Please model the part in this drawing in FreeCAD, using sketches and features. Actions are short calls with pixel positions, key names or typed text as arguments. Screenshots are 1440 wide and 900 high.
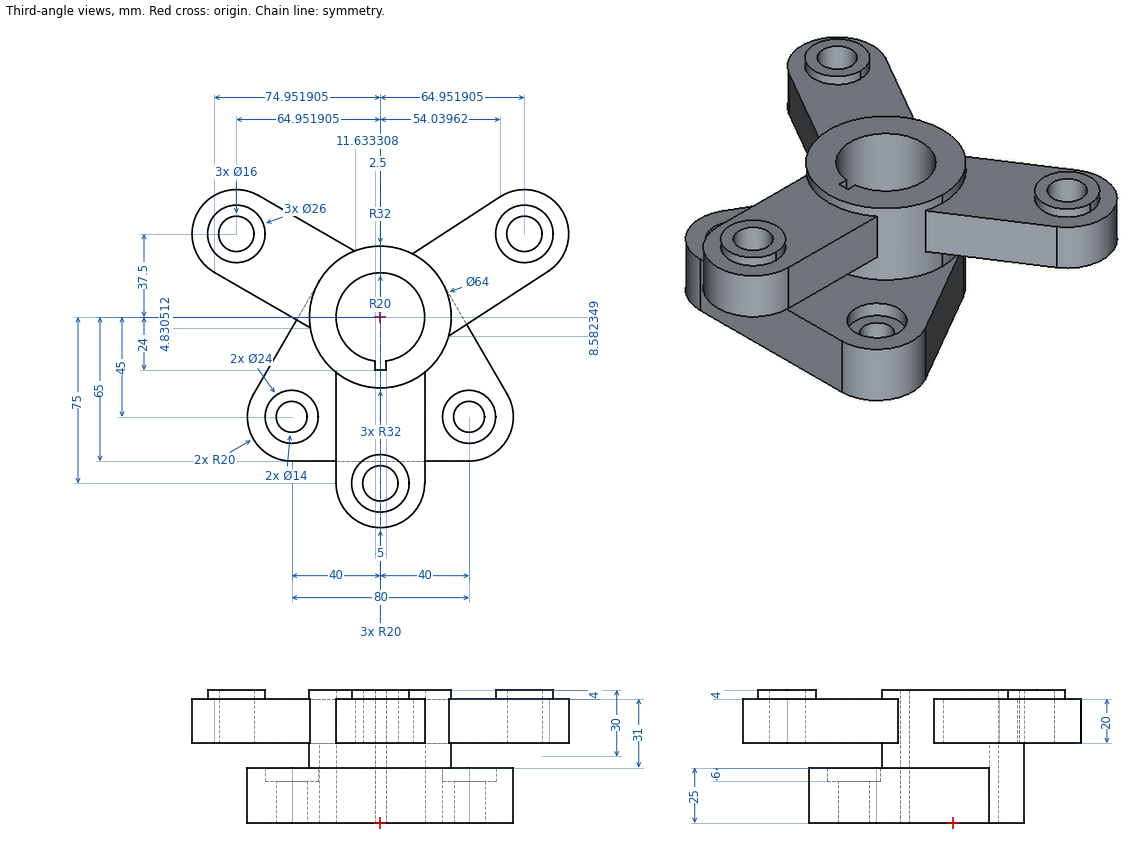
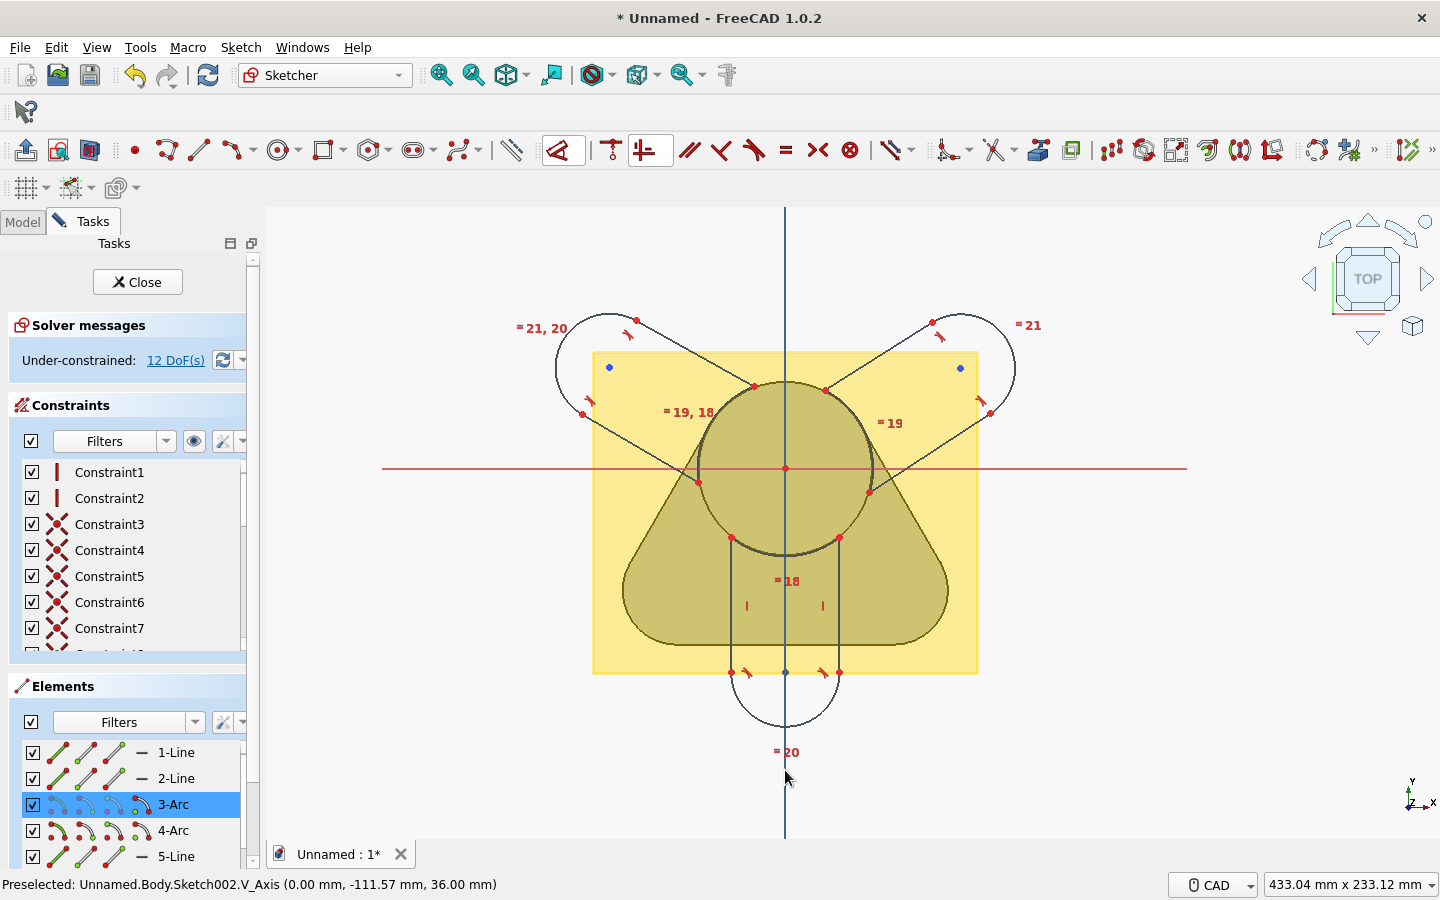
click(612, 150)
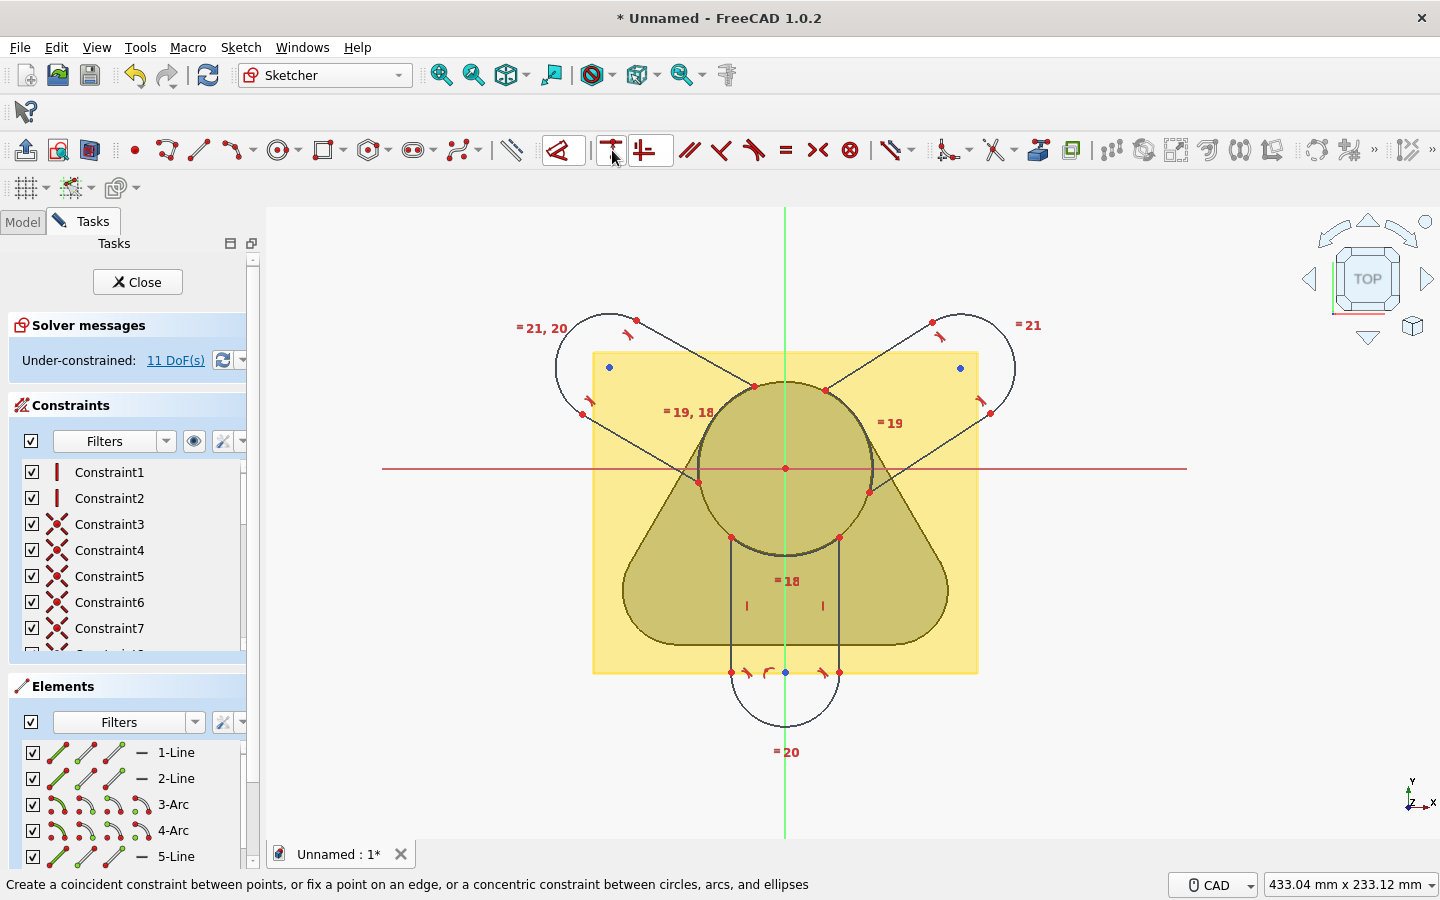
click(610, 368)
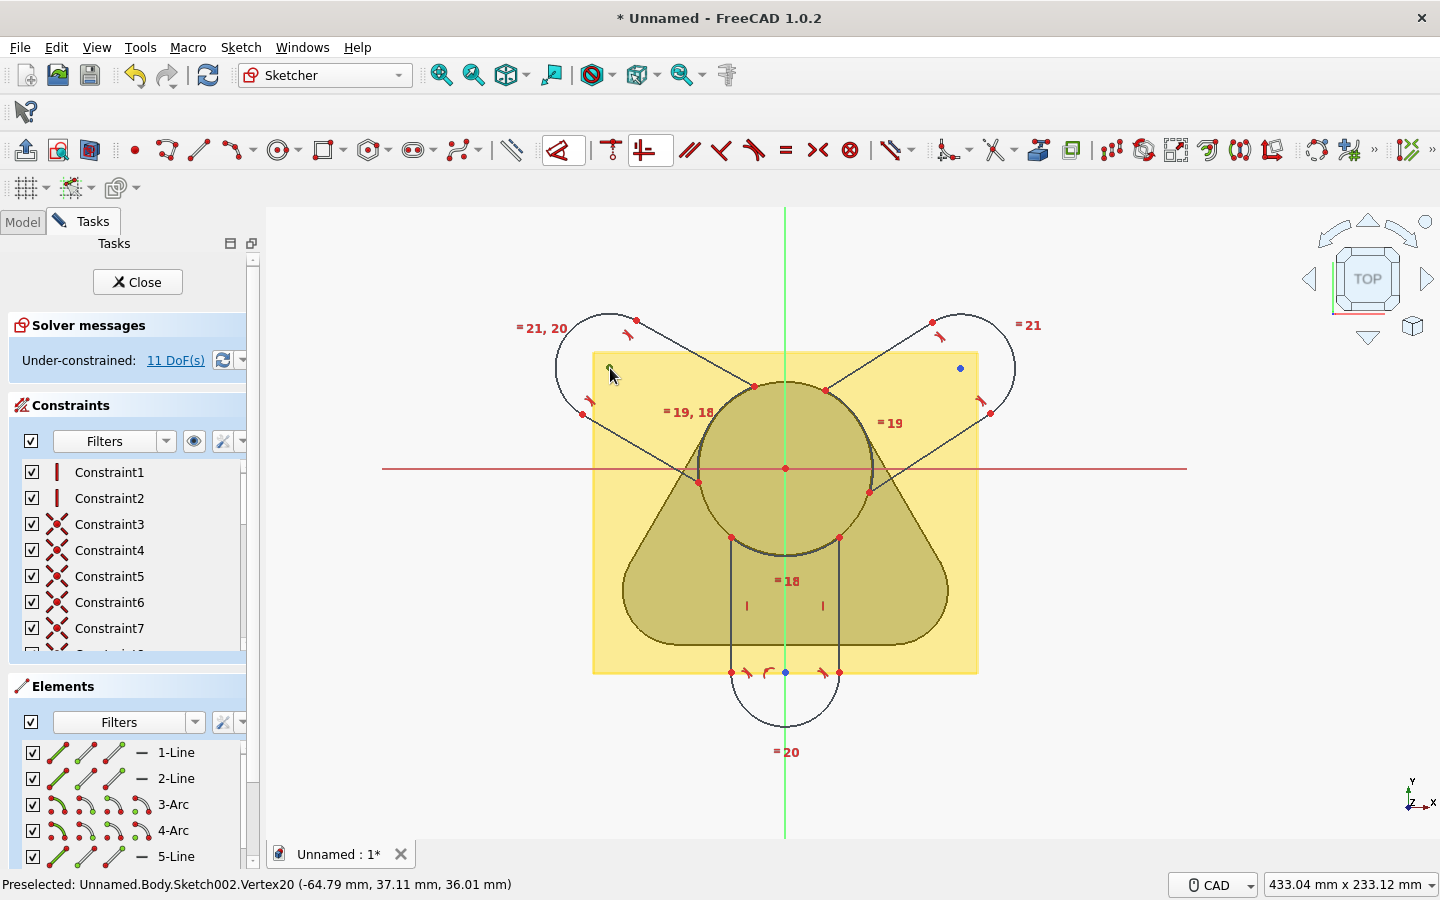
click(961, 368)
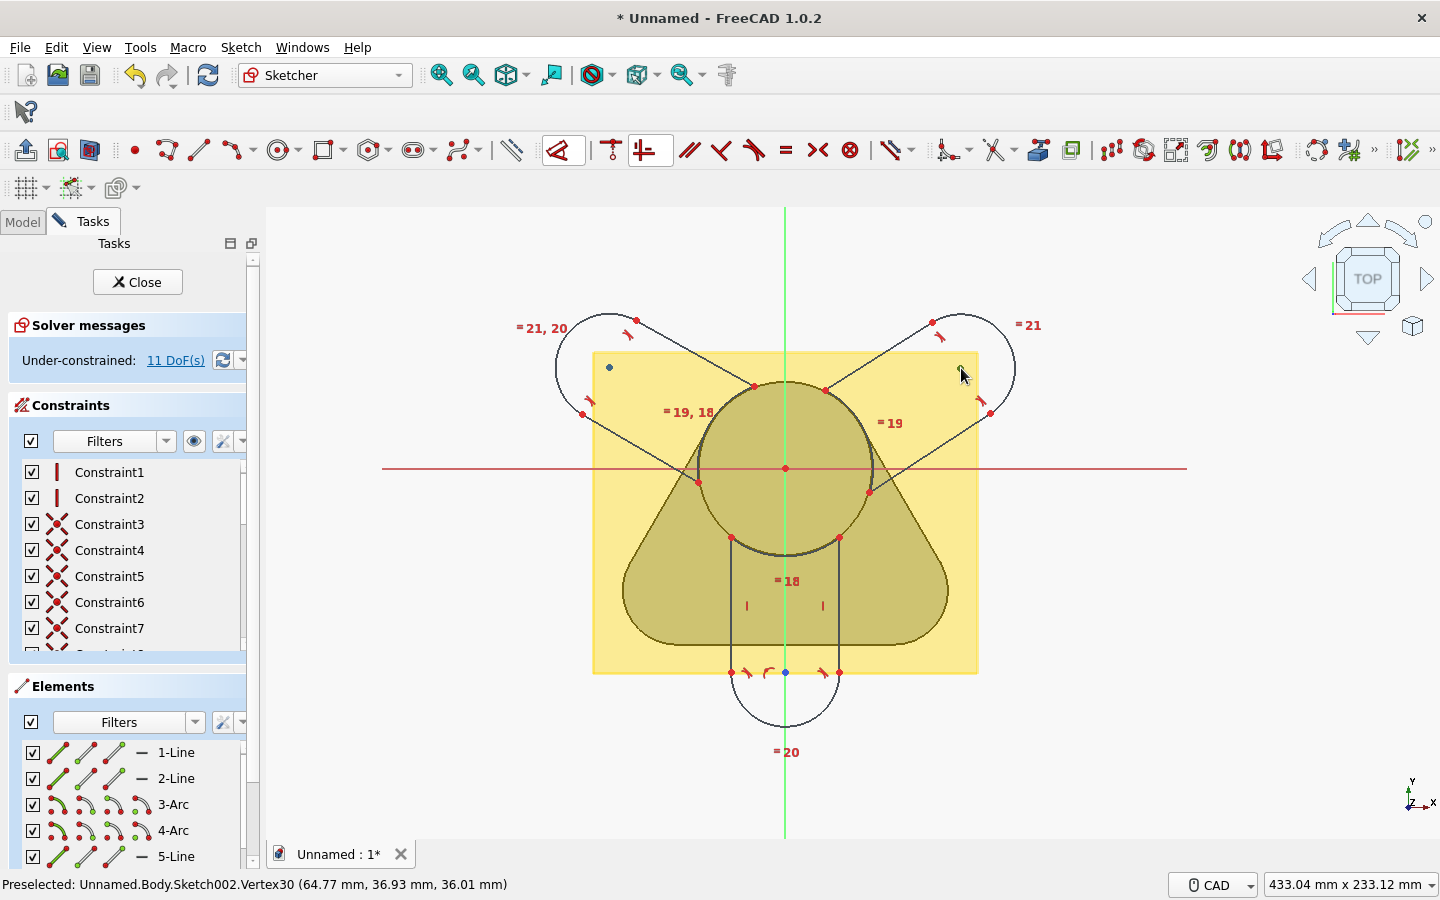
click(785, 770)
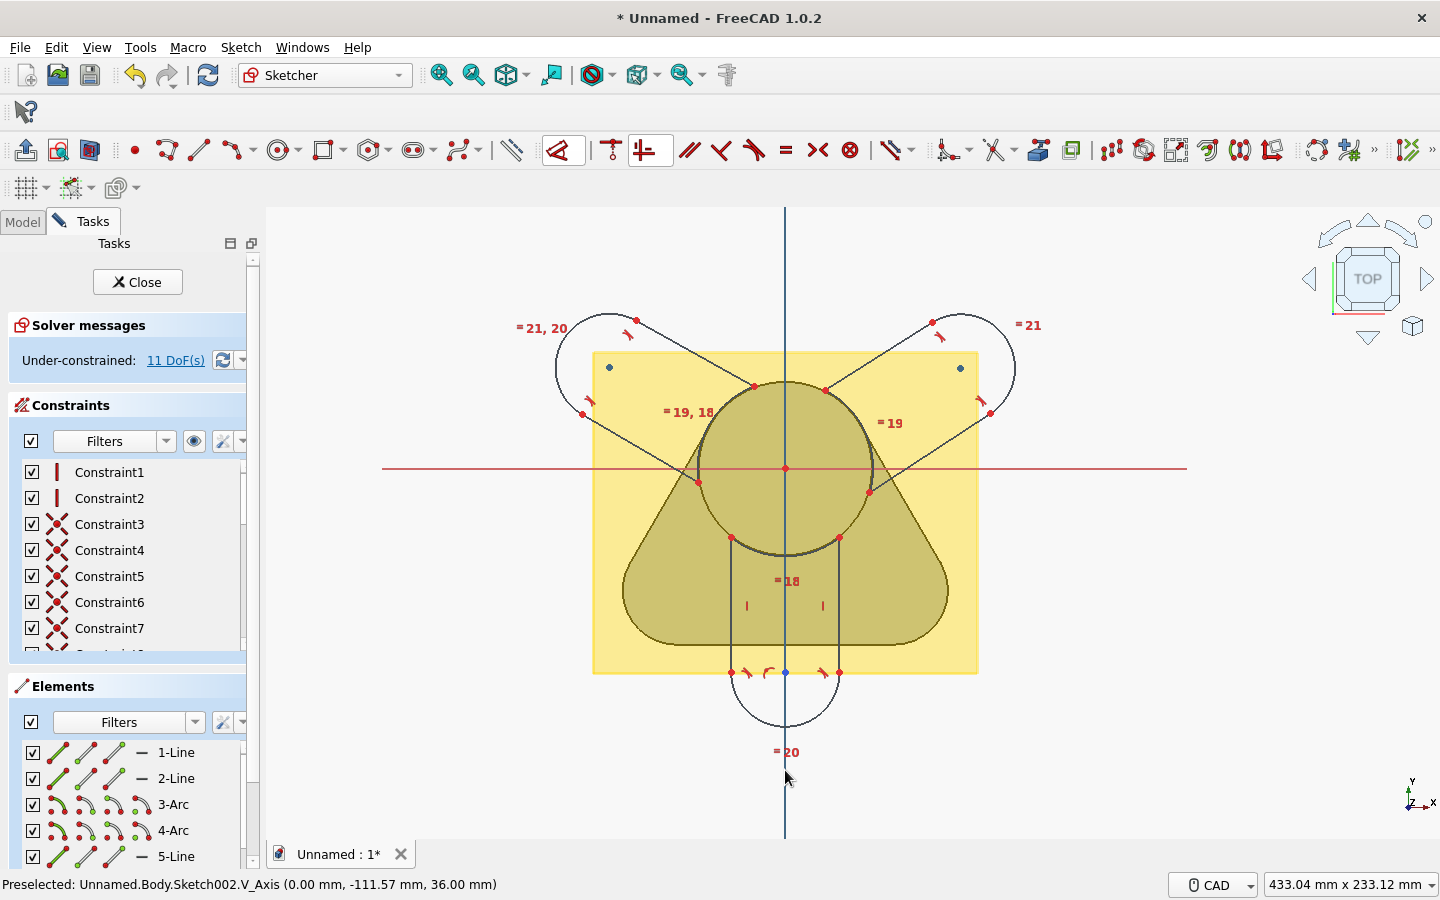
key(s)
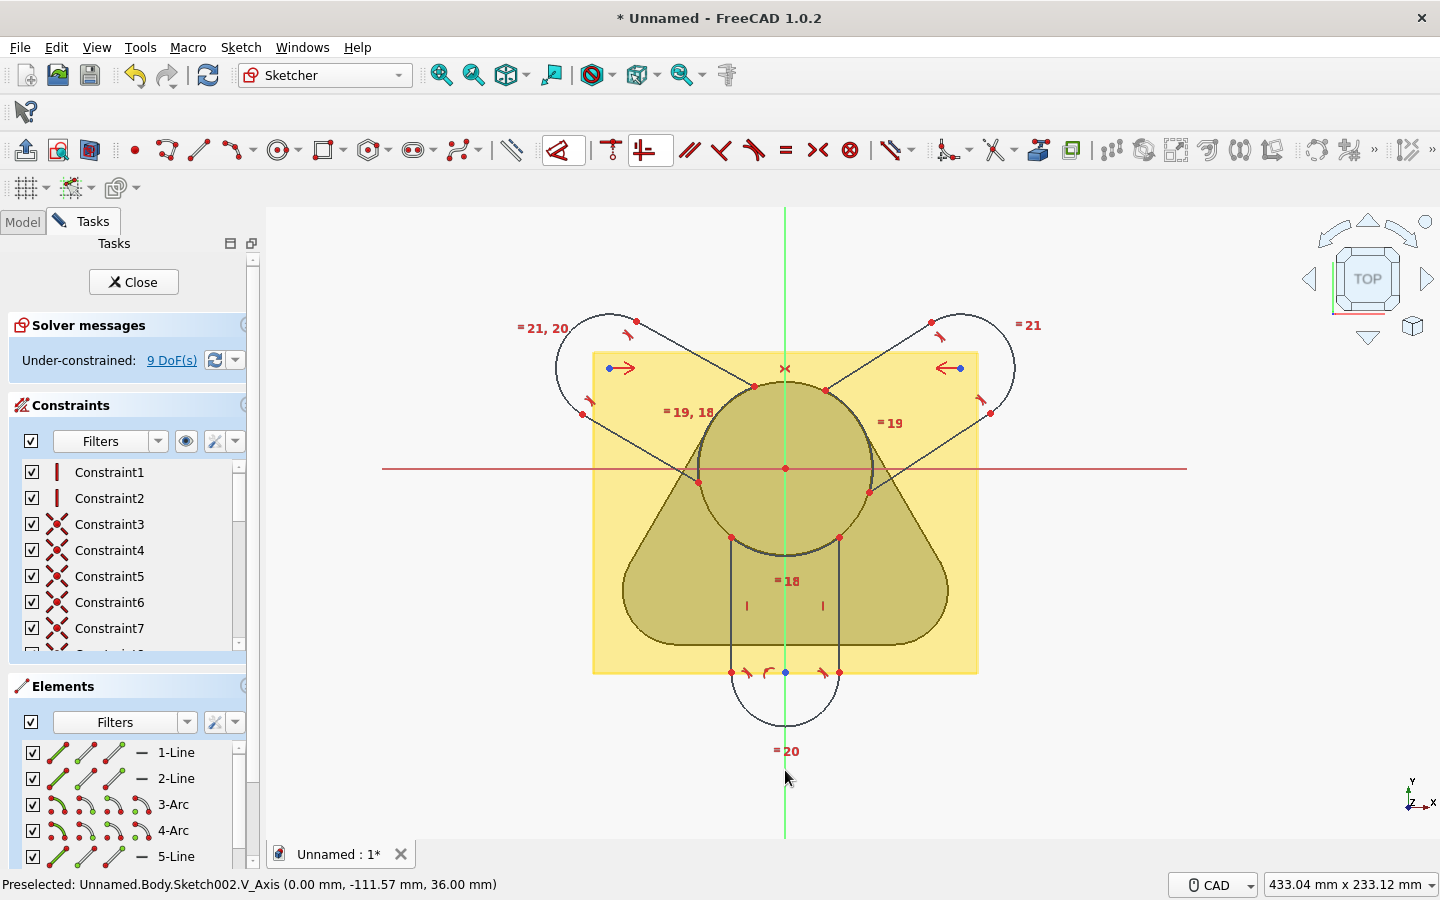
key(d)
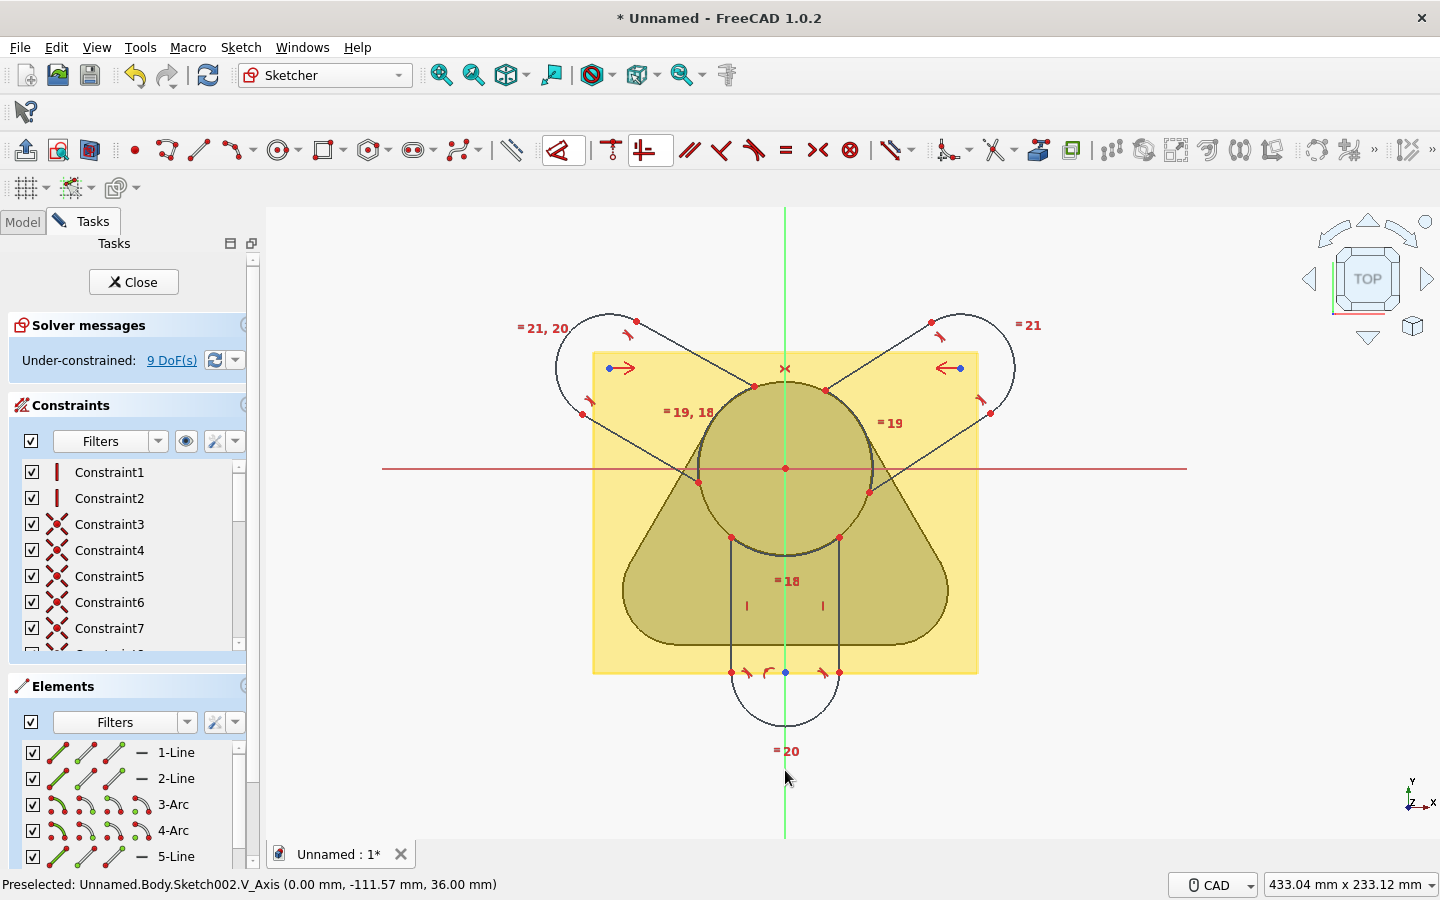
click(754, 716)
click(735, 742)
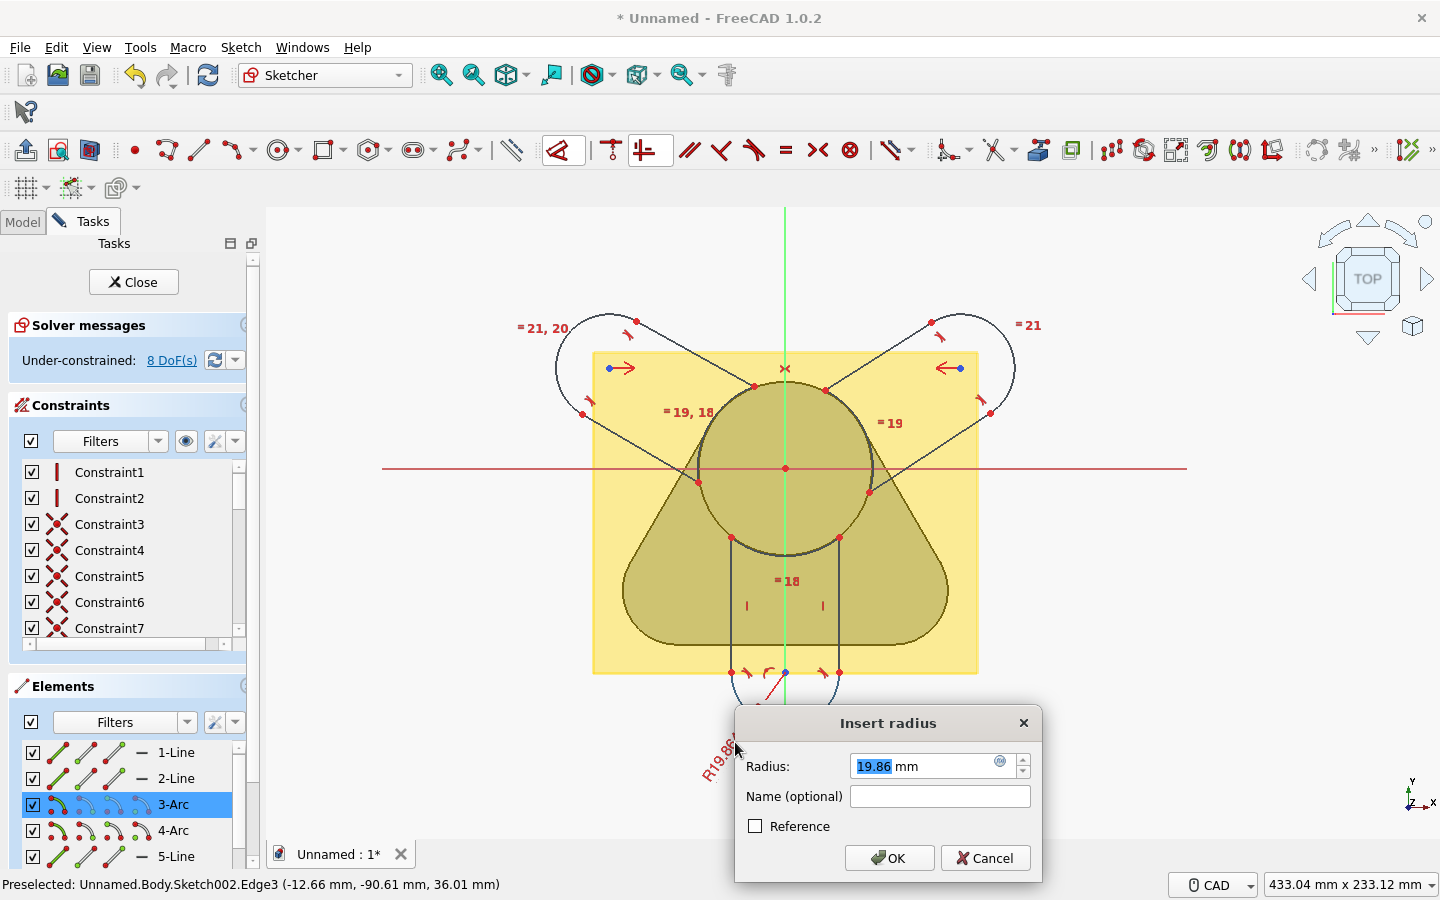
text(20)
key(Return)